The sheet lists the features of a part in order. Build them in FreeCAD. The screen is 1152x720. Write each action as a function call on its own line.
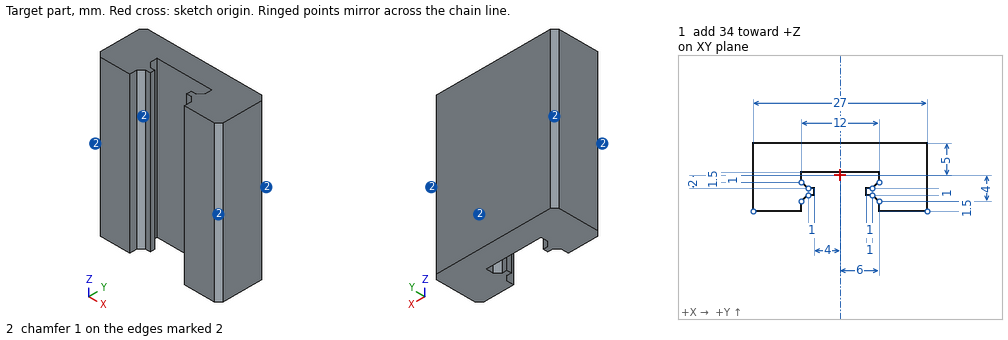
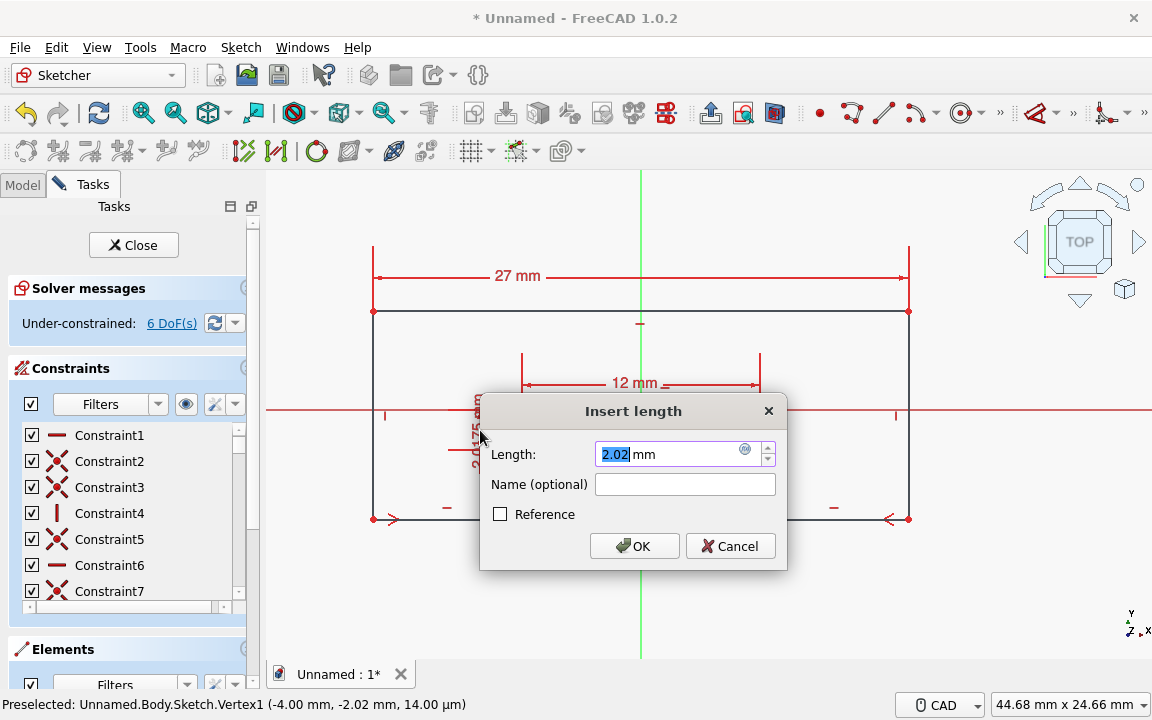
text(2)
key(Return)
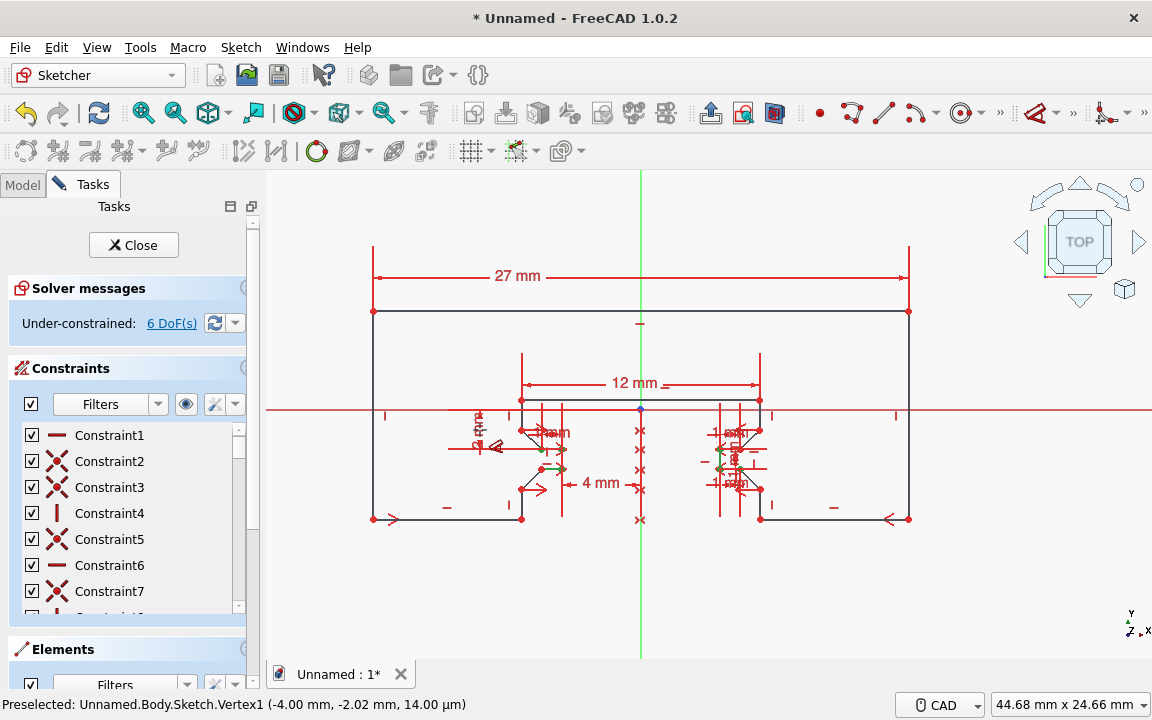
scroll(522, 430, up, 4)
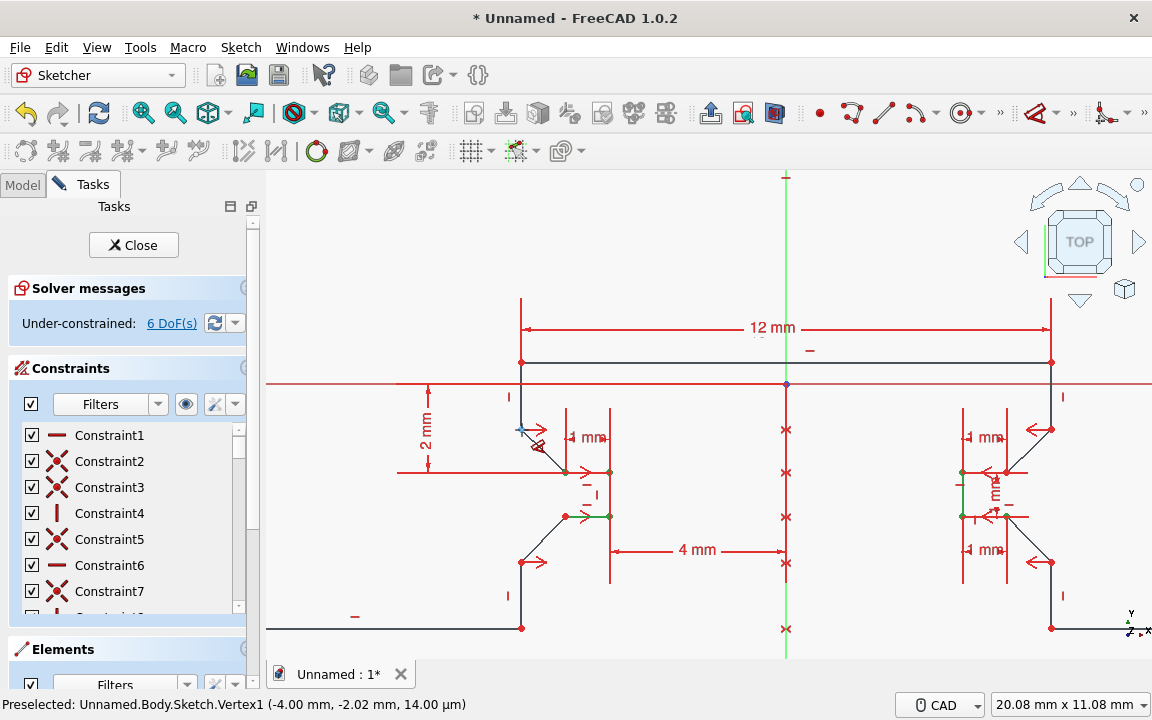
click(521, 430)
click(487, 407)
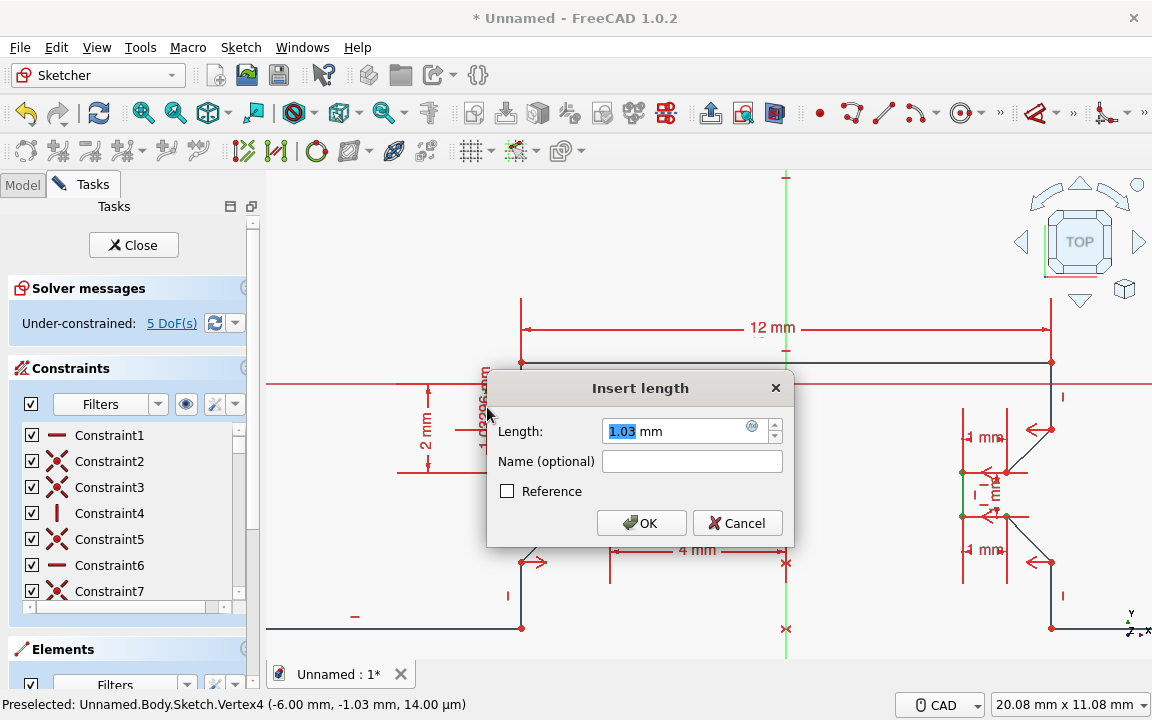
text(1)
key(Return)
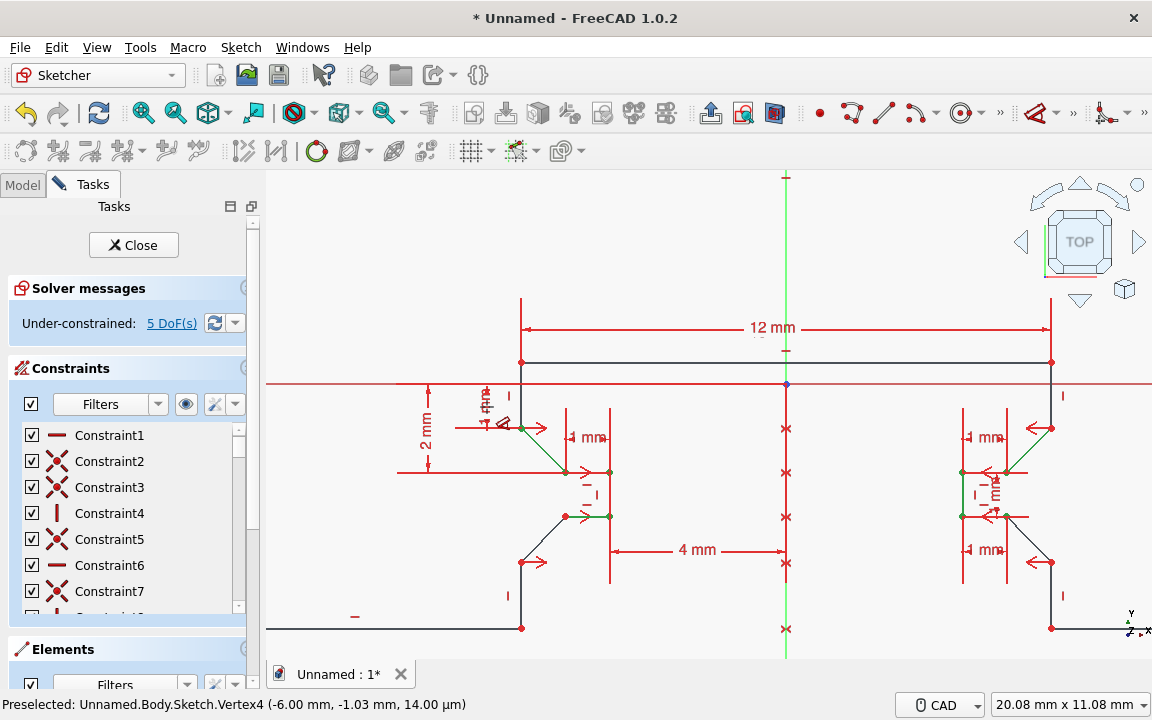
scroll(522, 430, down, 4)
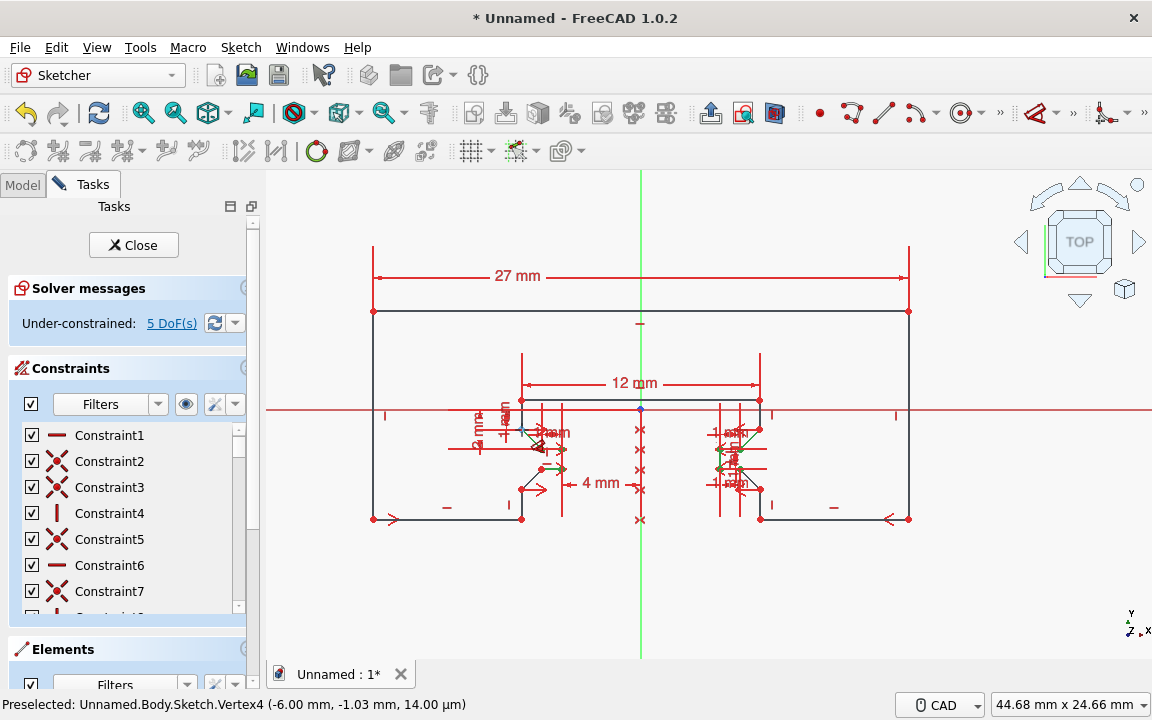
click(760, 490)
click(700, 524)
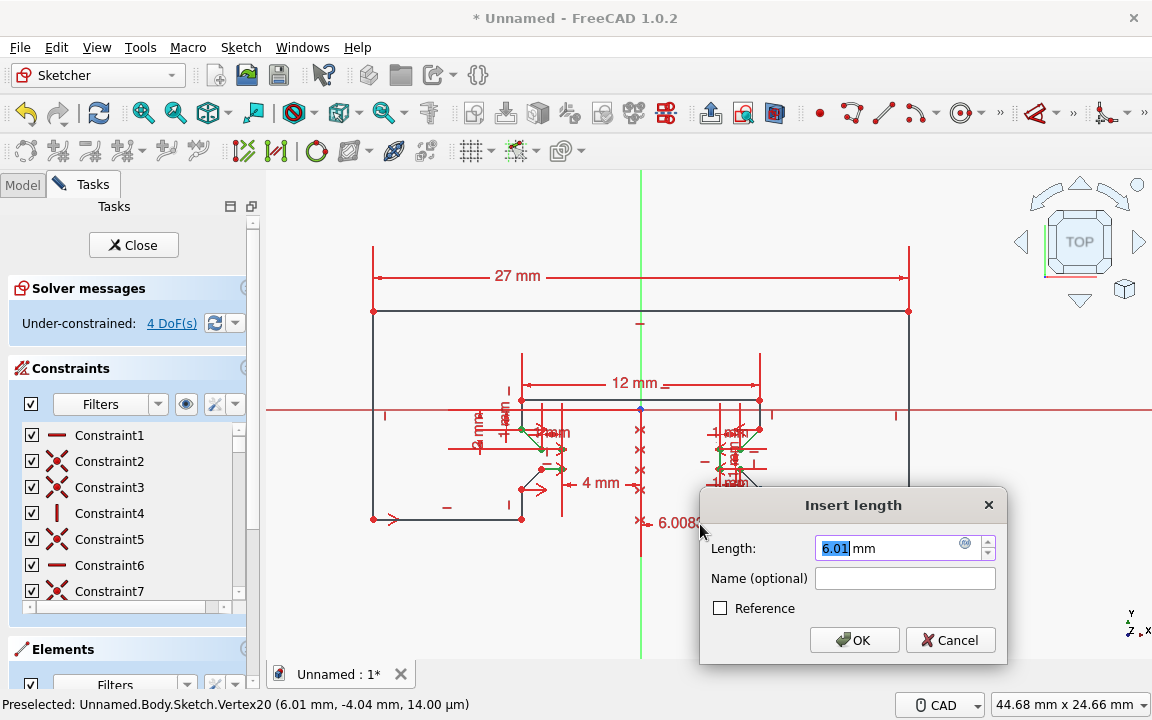
text(6)
key(Return)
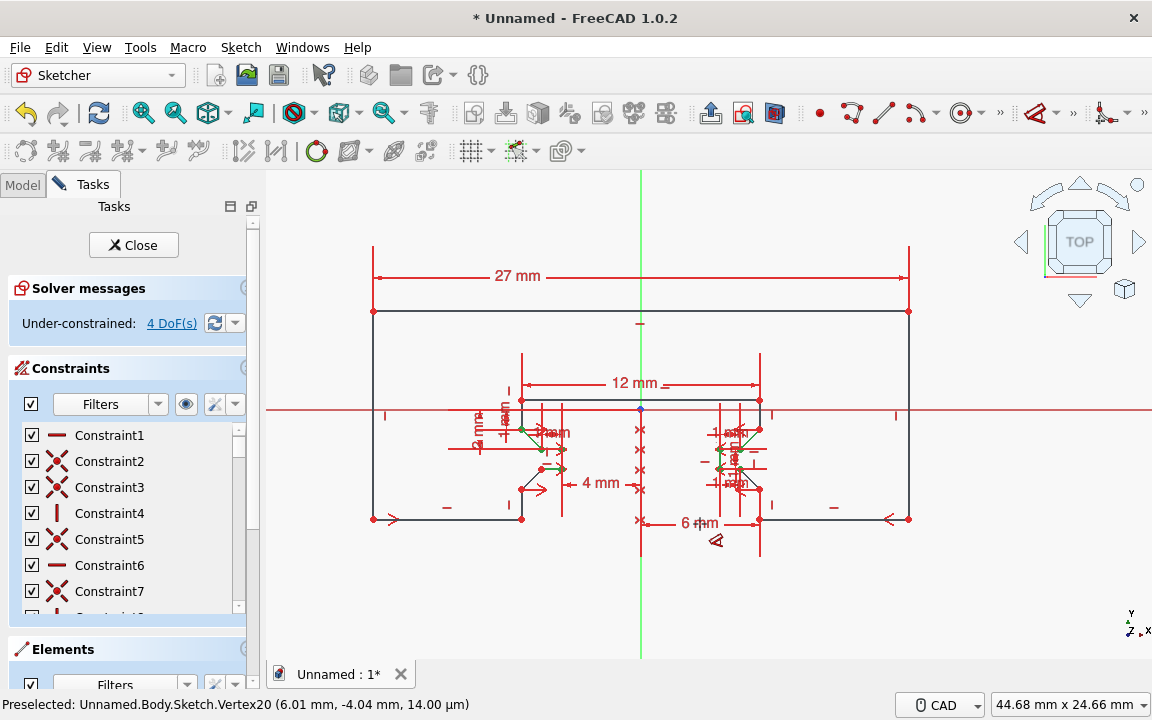
click(760, 490)
click(818, 450)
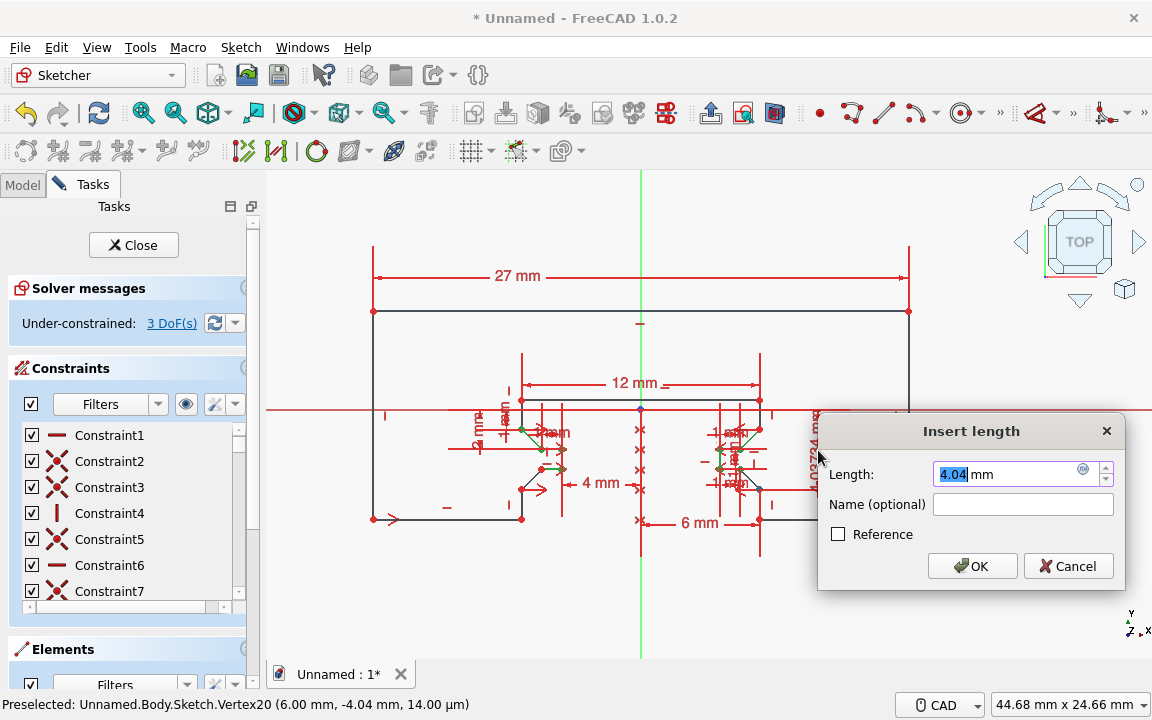
text(4)
key(Return)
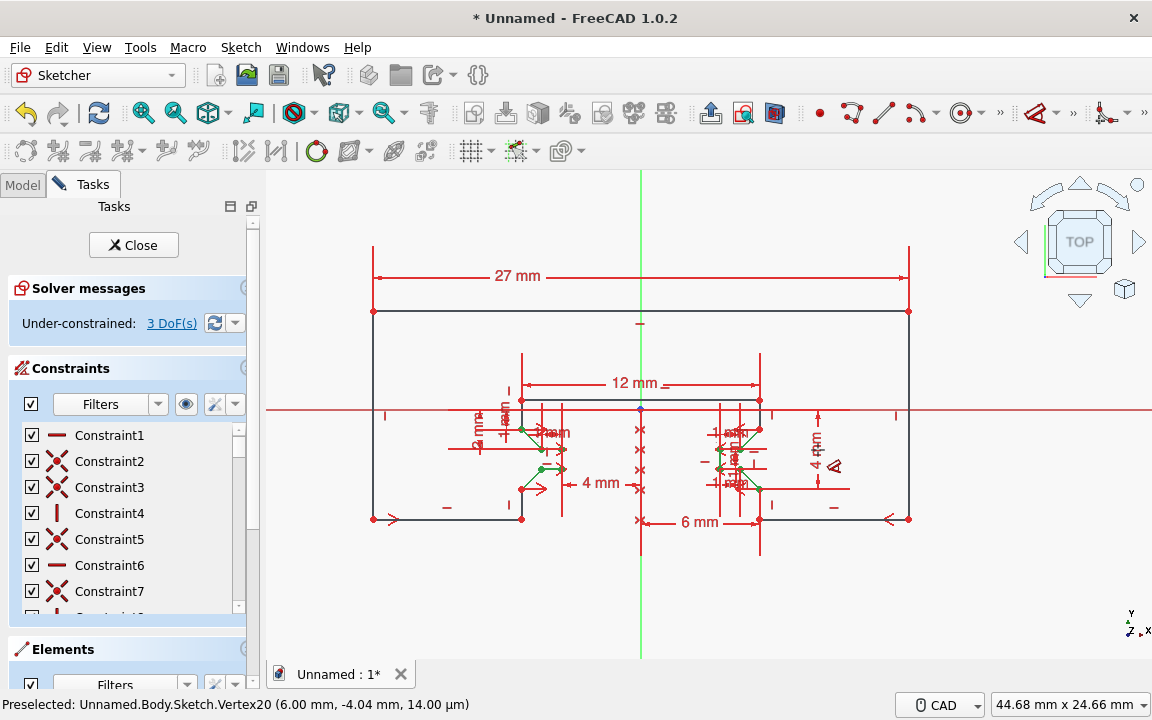
click(909, 311)
click(943, 361)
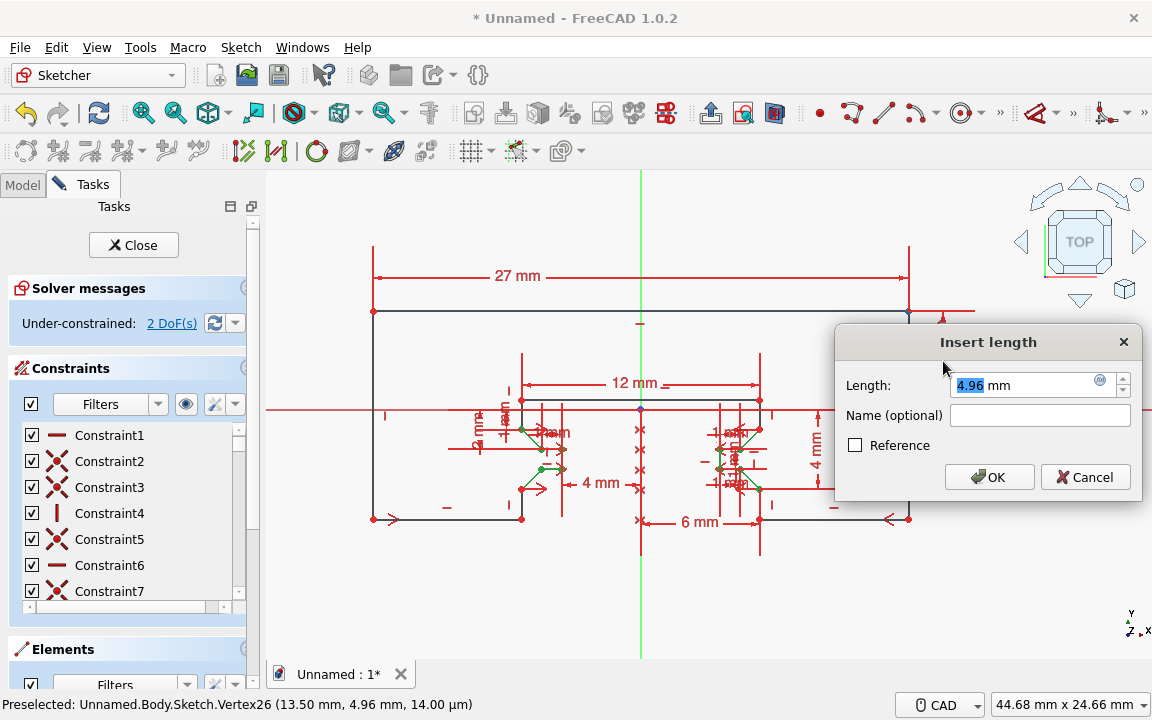
text(5)
key(Return)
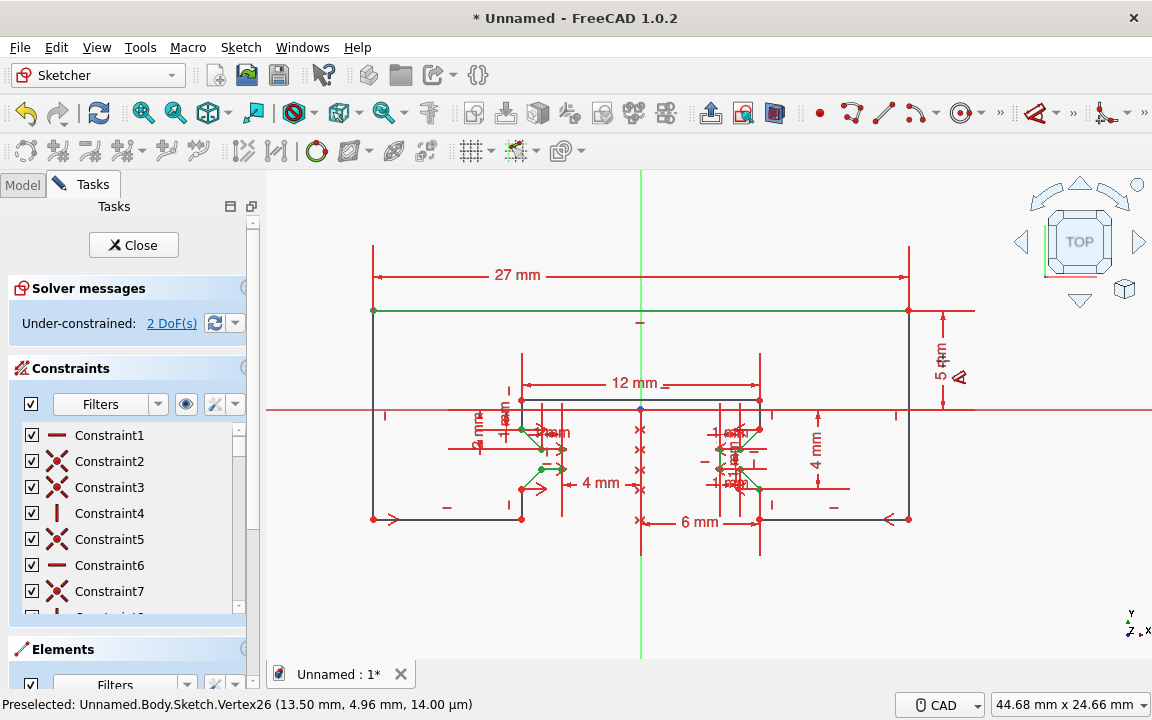
scroll(522, 412, up, 2)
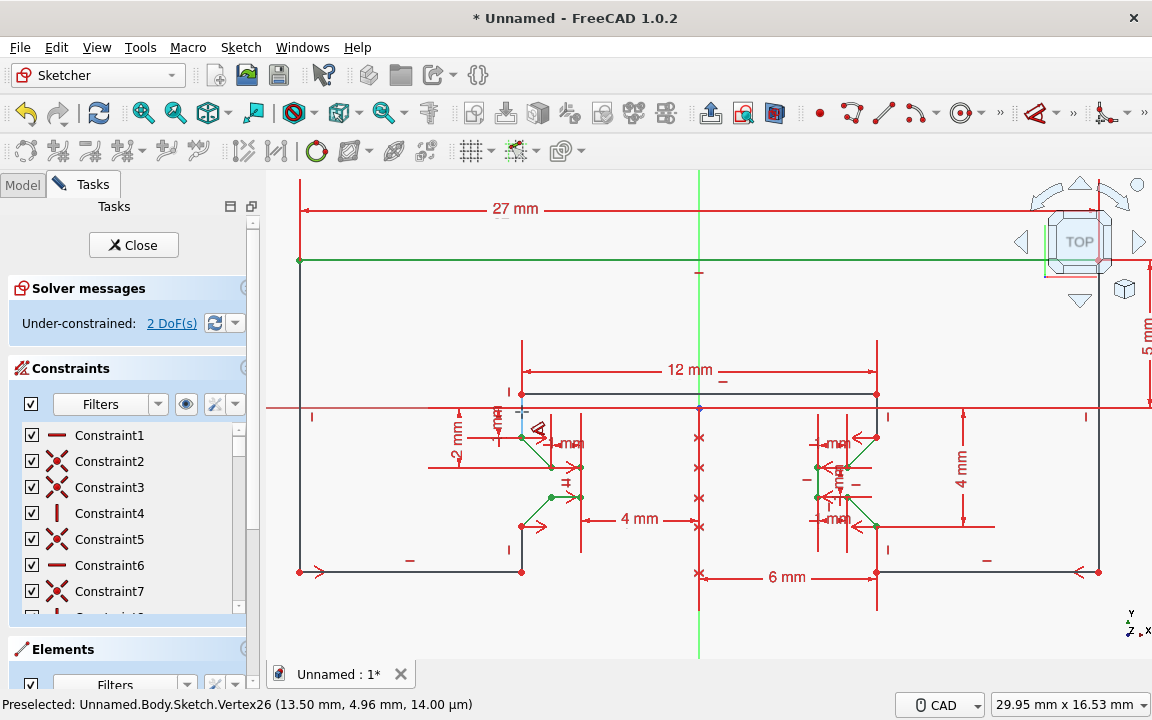
click(522, 412)
click(652, 426)